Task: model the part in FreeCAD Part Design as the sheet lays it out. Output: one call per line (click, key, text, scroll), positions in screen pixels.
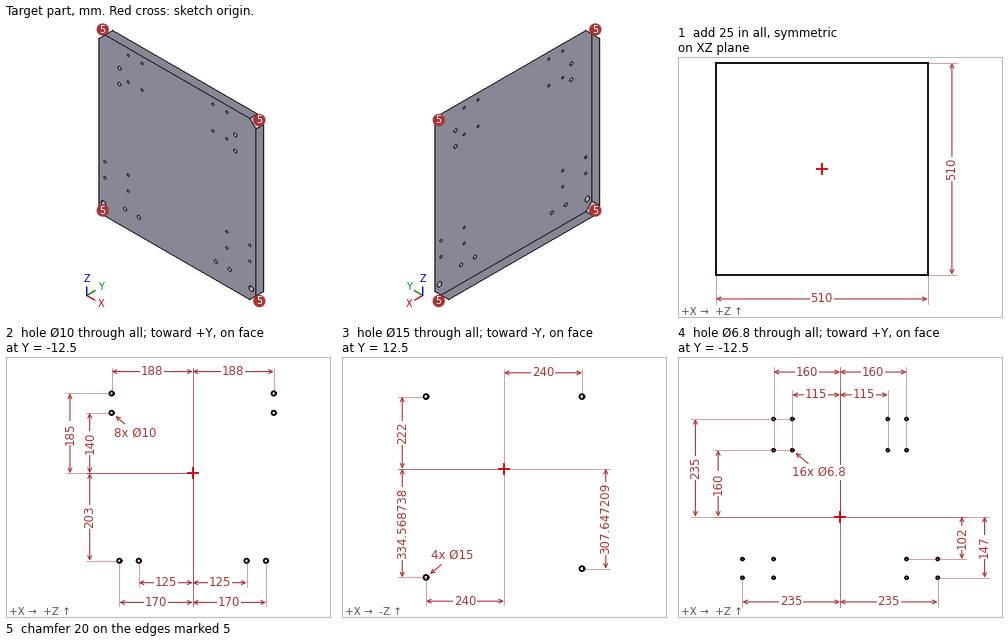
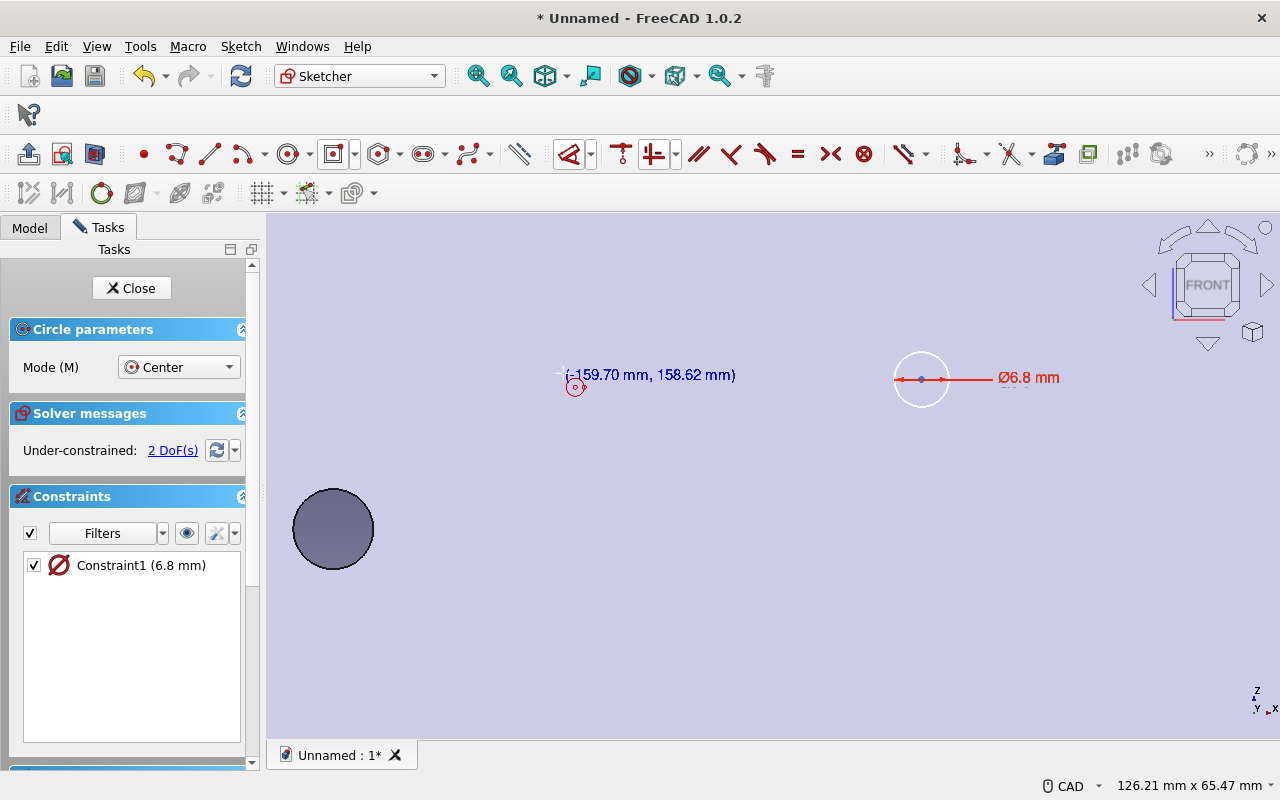
scroll(563, 373, down, 11)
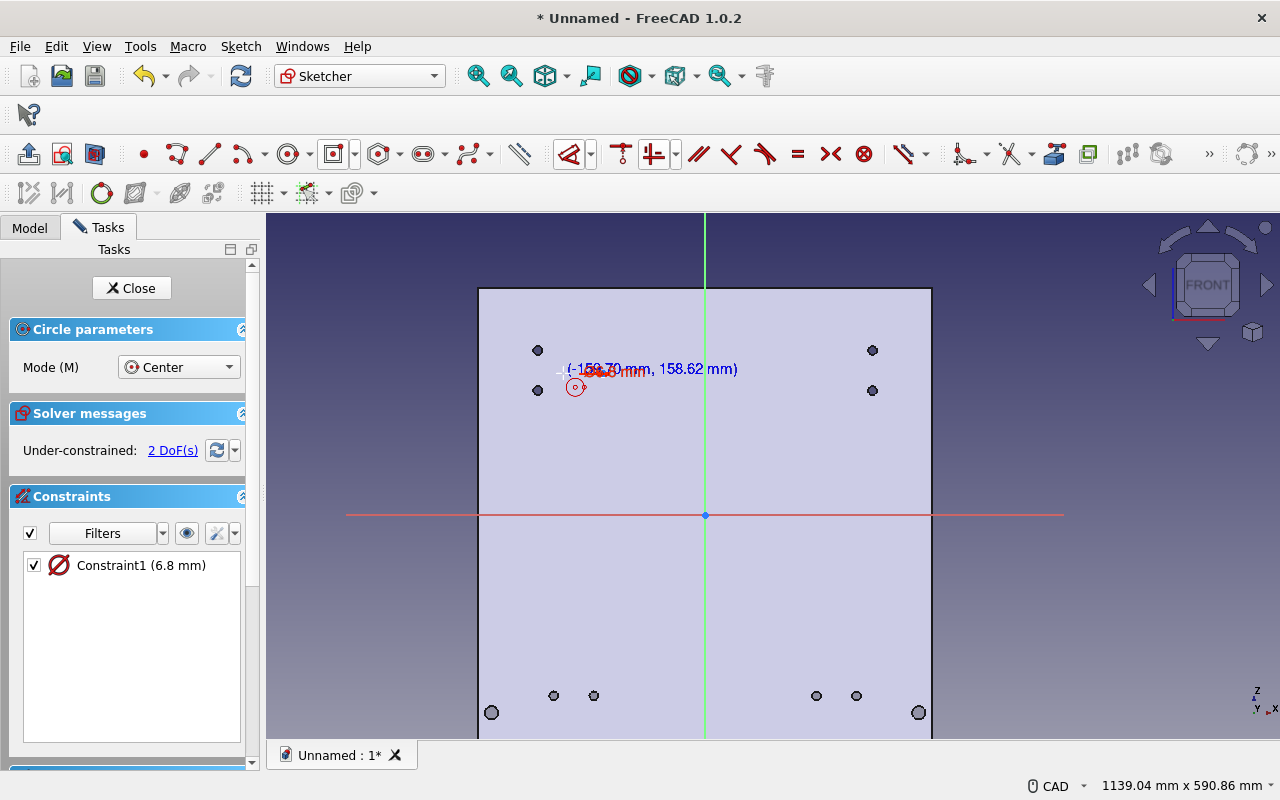
click(563, 373)
move(565, 371)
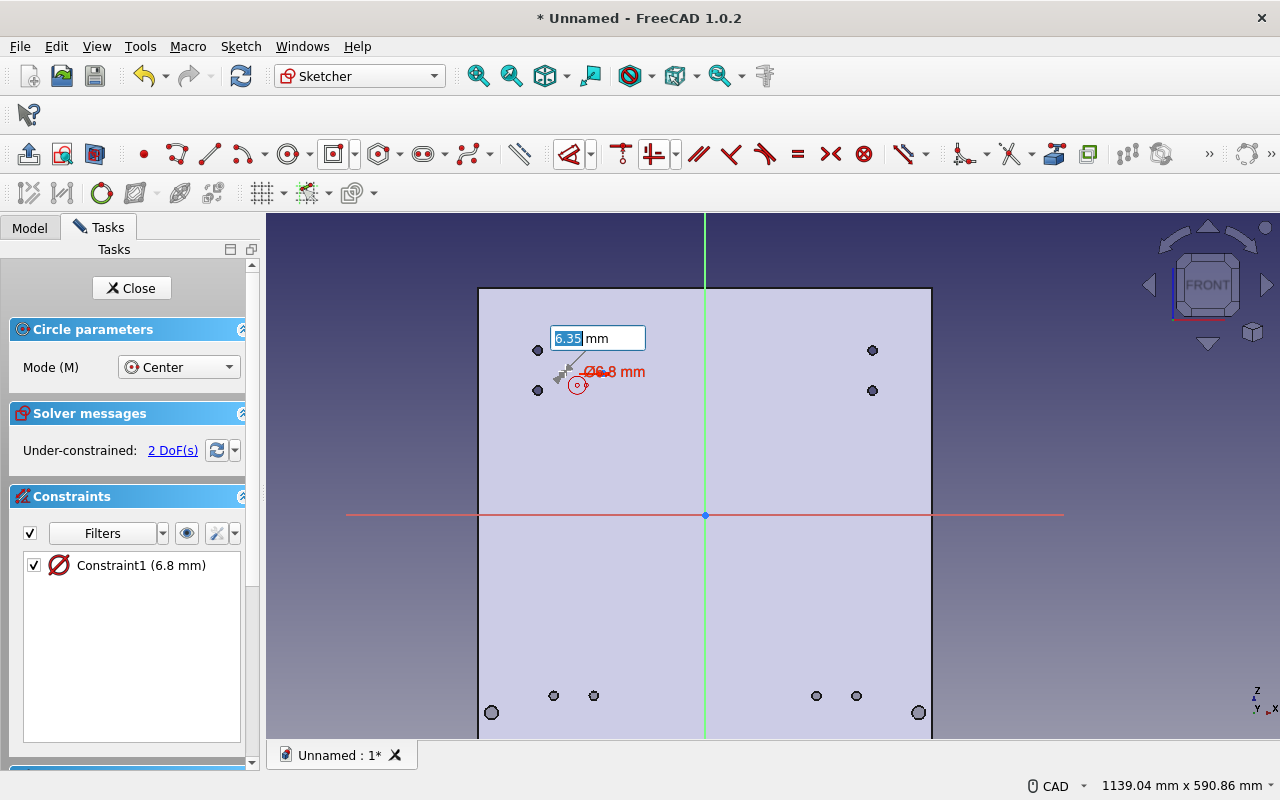
text(6.8)
key(Return)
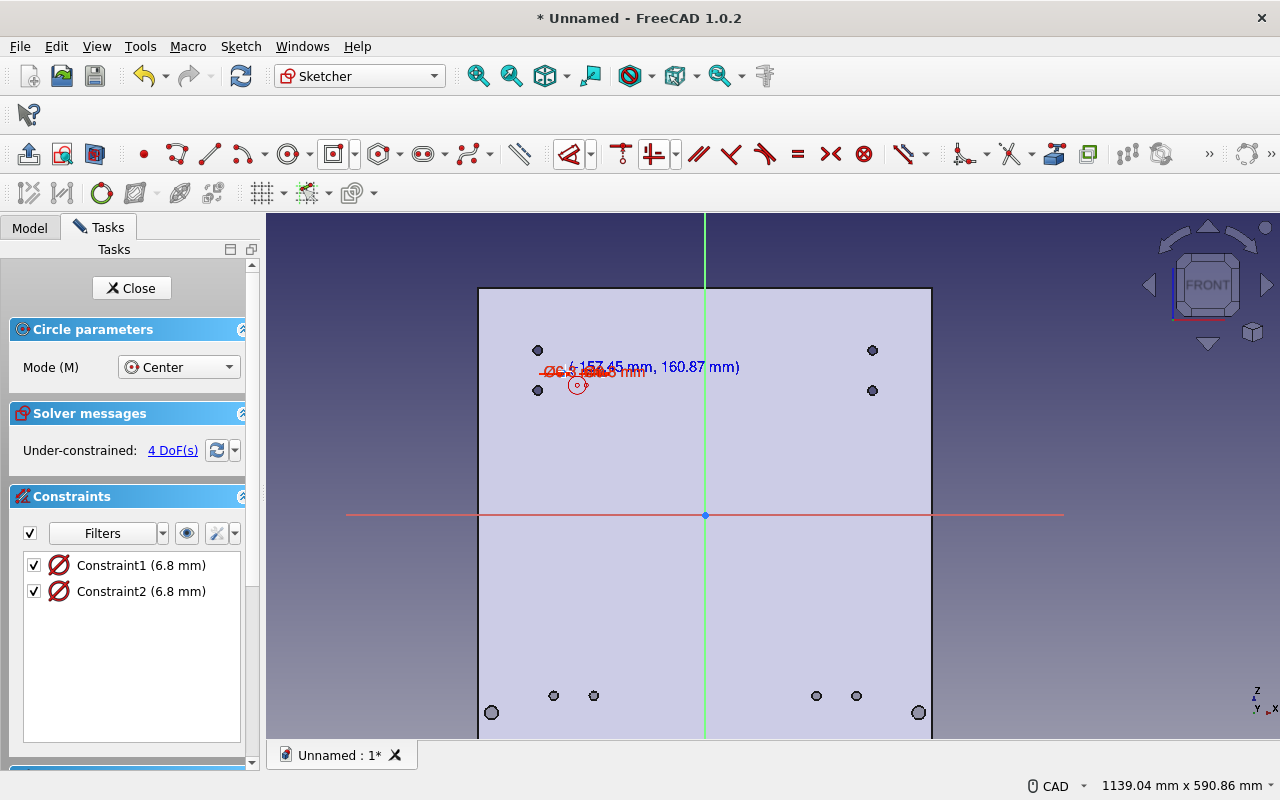
scroll(603, 306, up, 11)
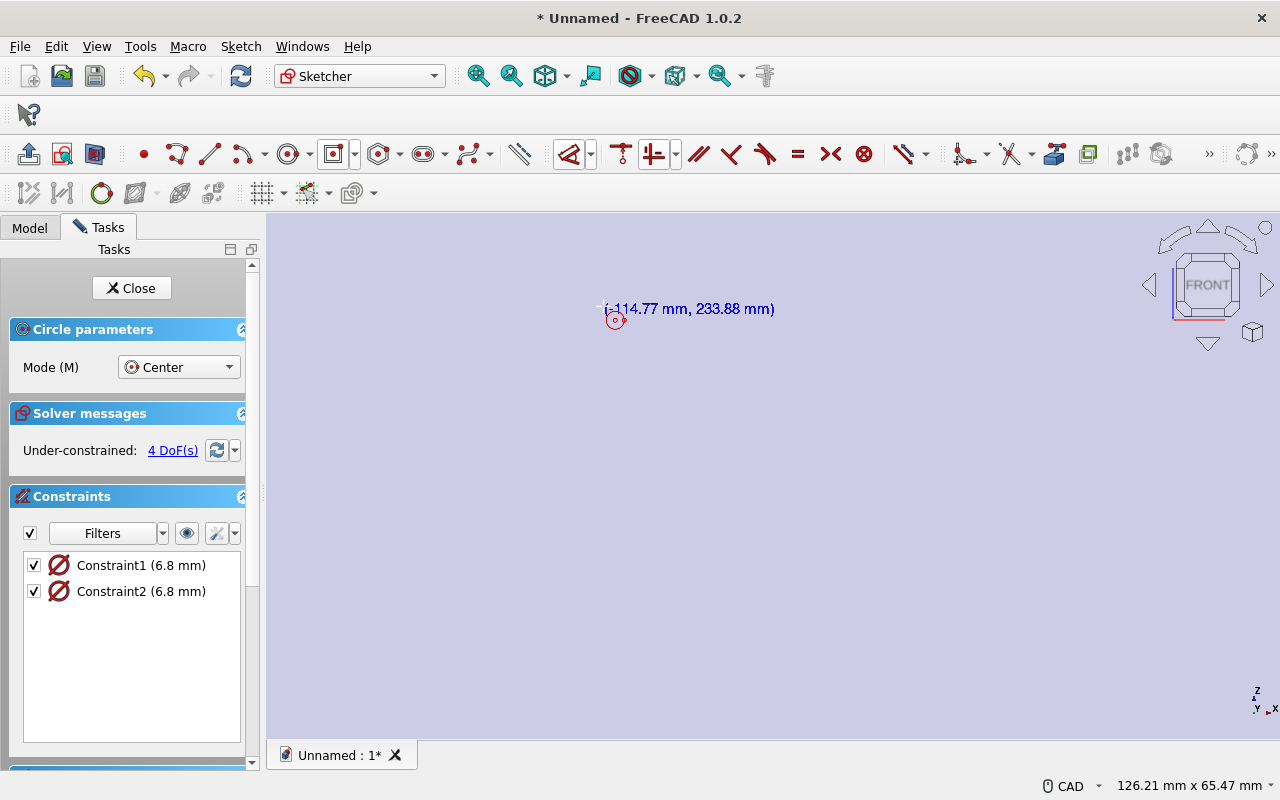
scroll(603, 306, down, 11)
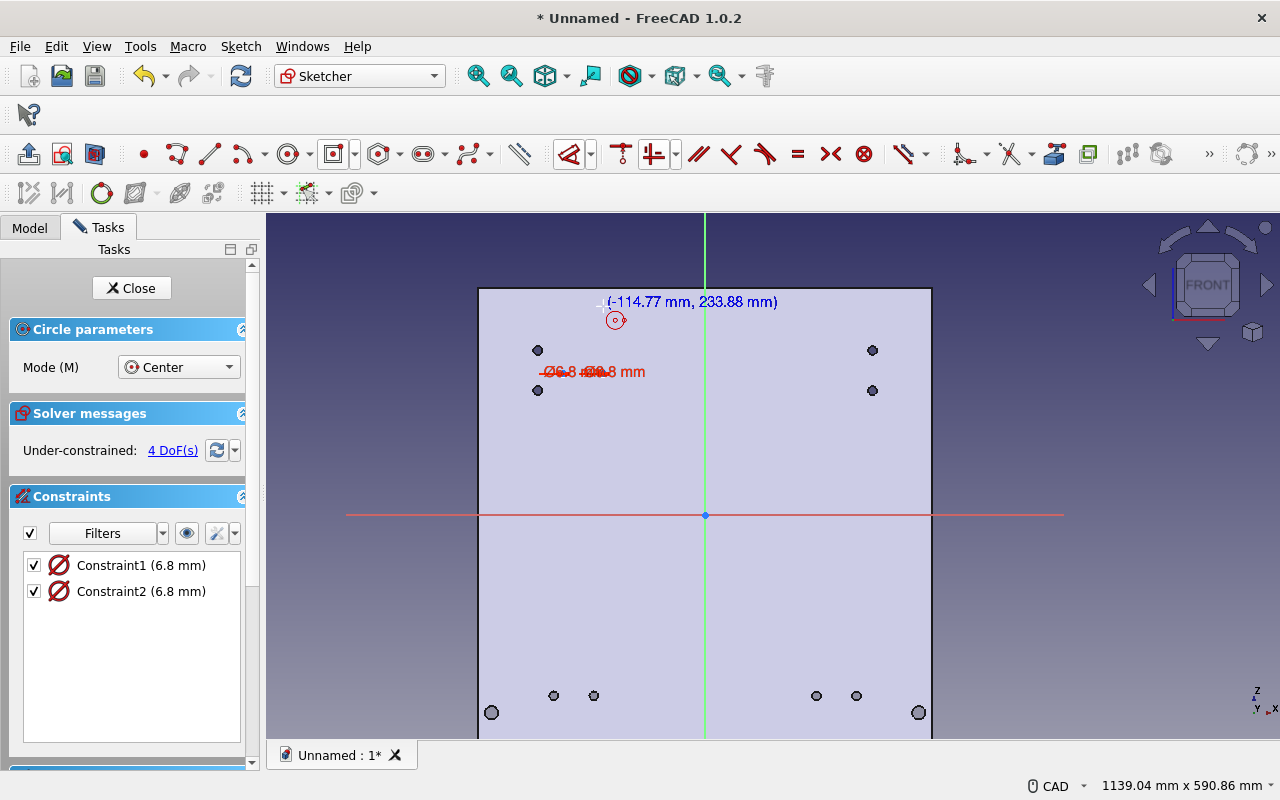
click(603, 306)
move(605, 304)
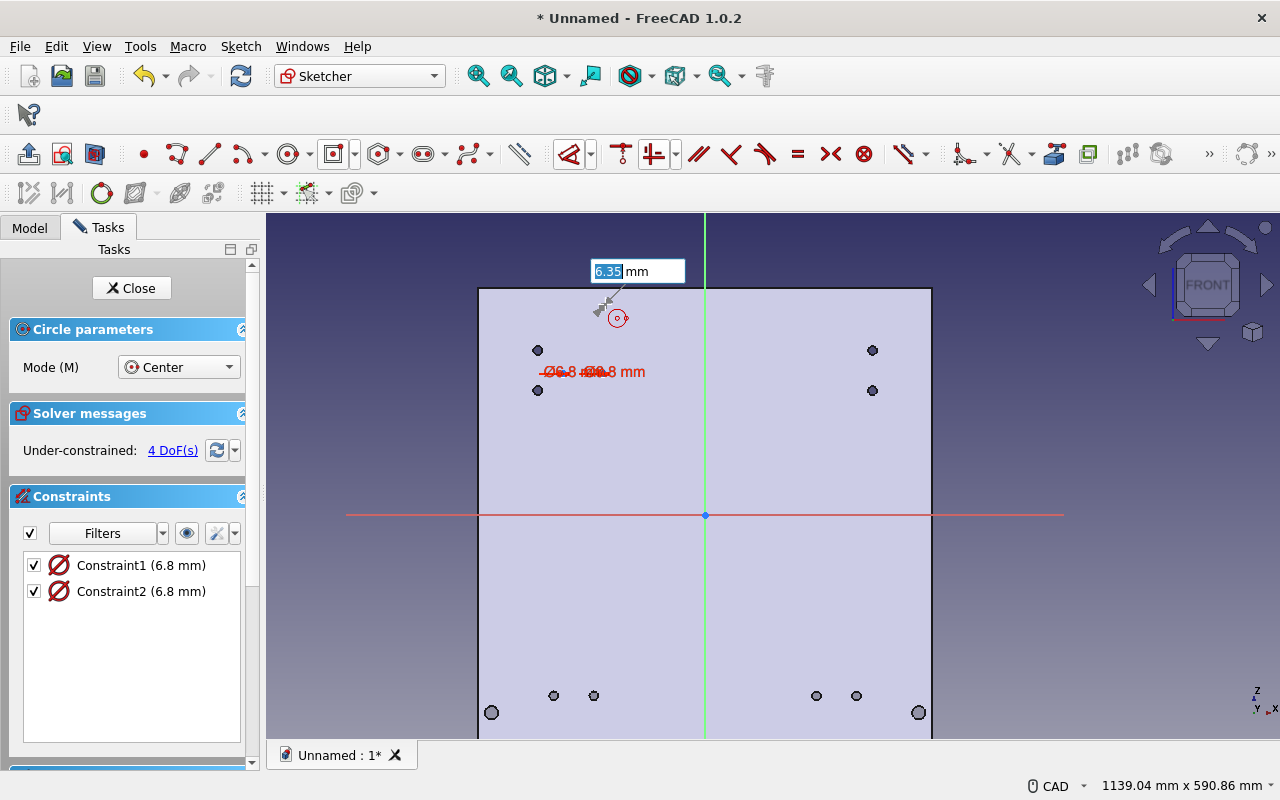
text(6.8)
key(Return)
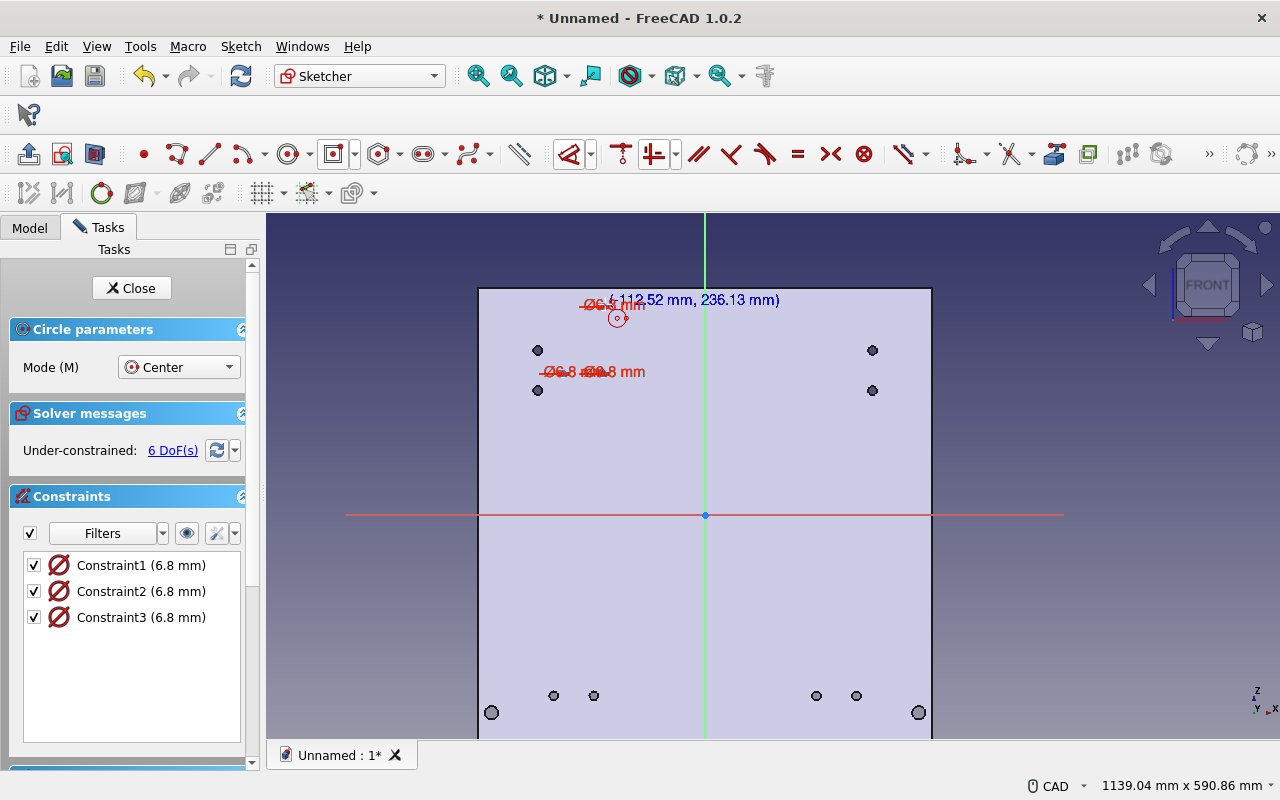
scroll(563, 306, up, 11)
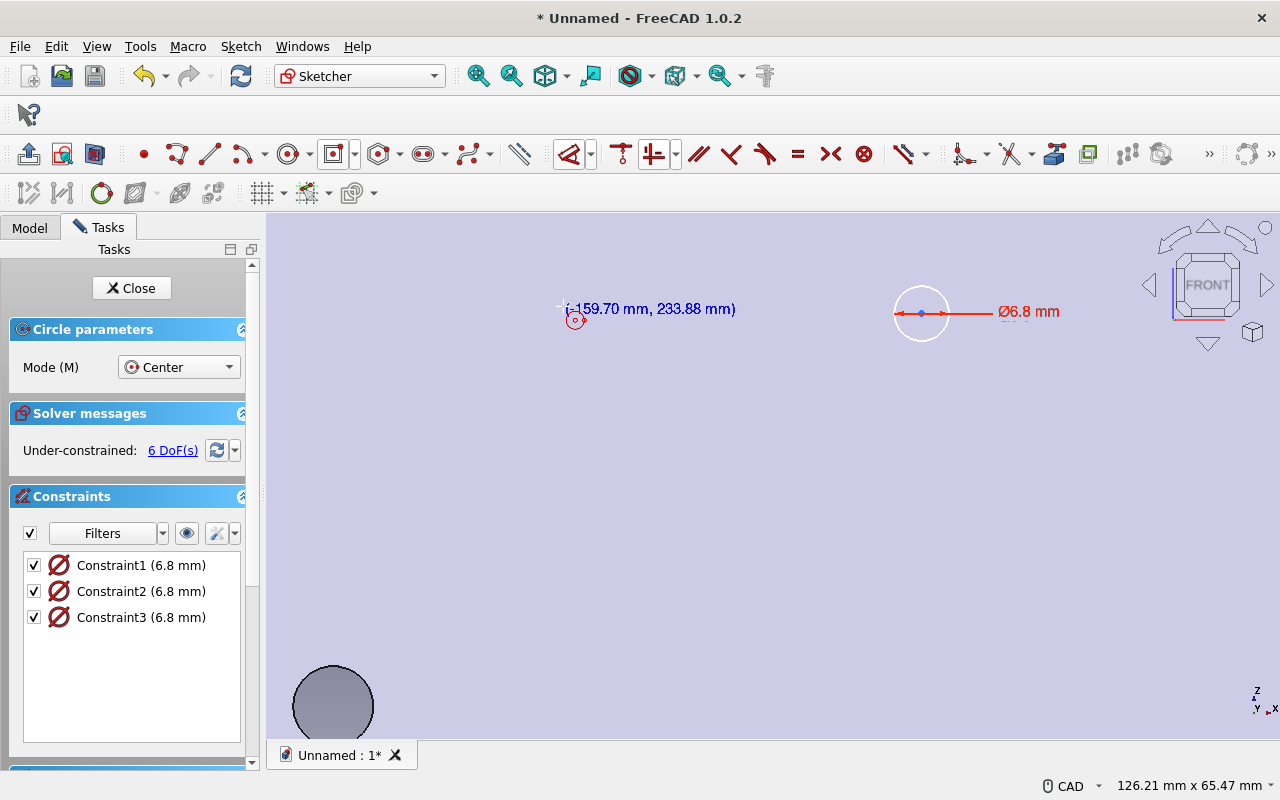
scroll(563, 306, down, 11)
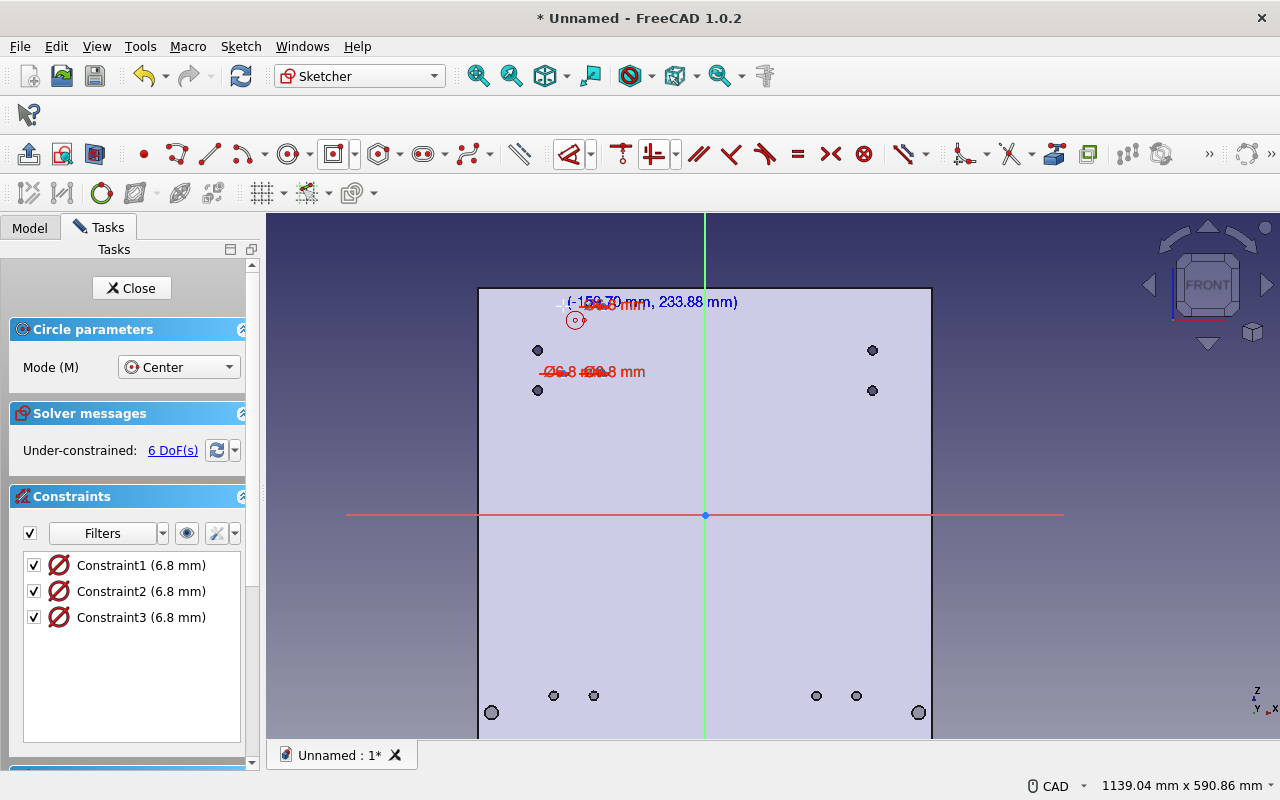
click(563, 306)
move(565, 304)